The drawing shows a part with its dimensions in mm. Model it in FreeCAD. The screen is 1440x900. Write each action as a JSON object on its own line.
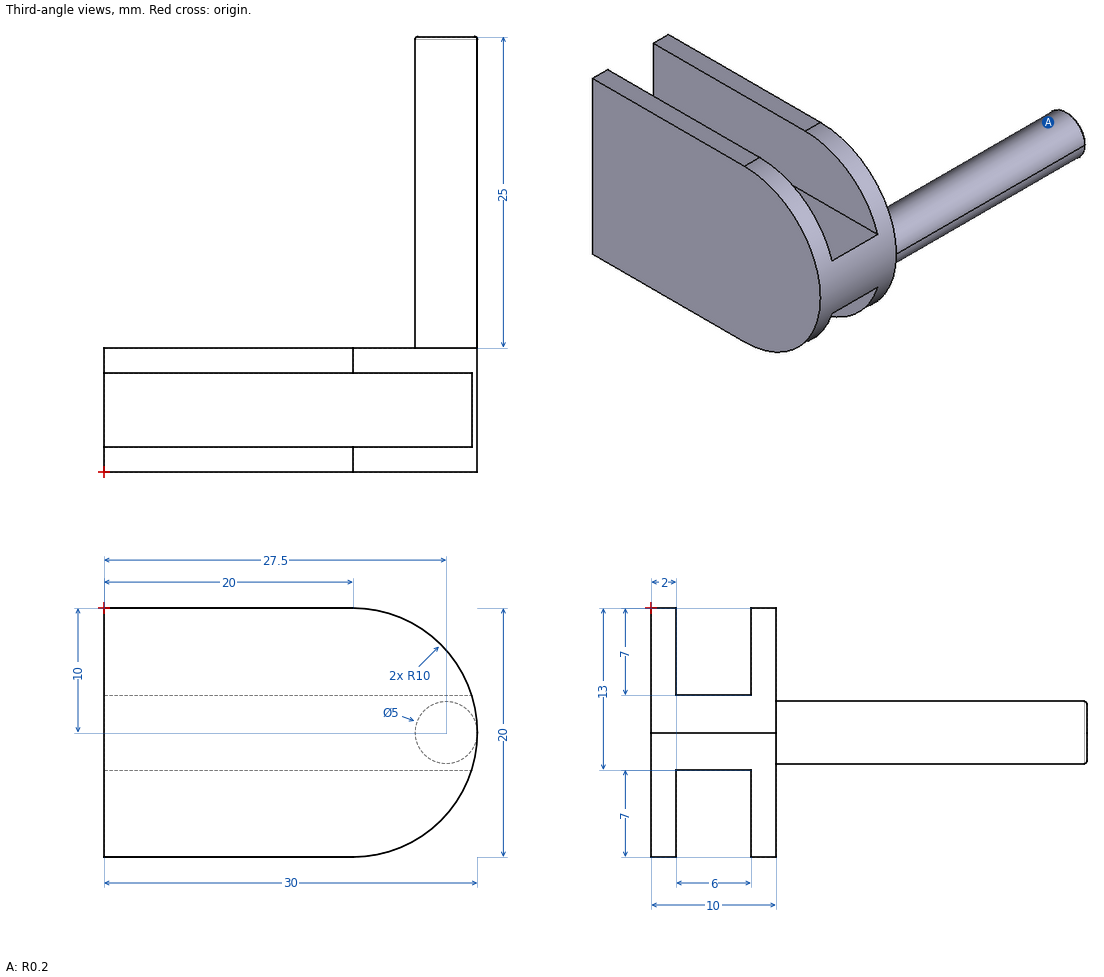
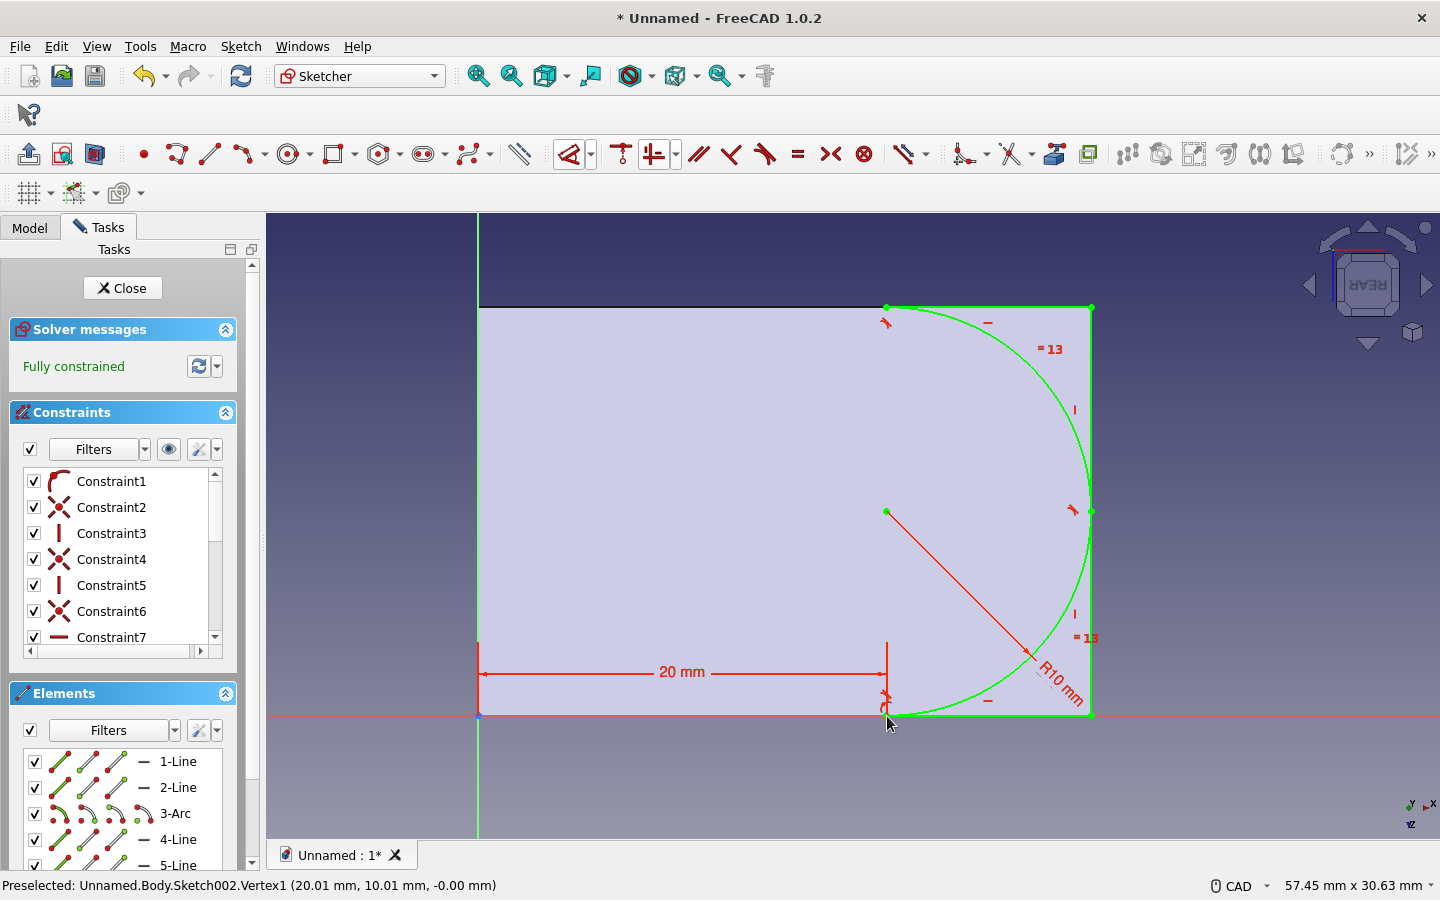
{"action": "left_click", "coordinate": [123, 288]}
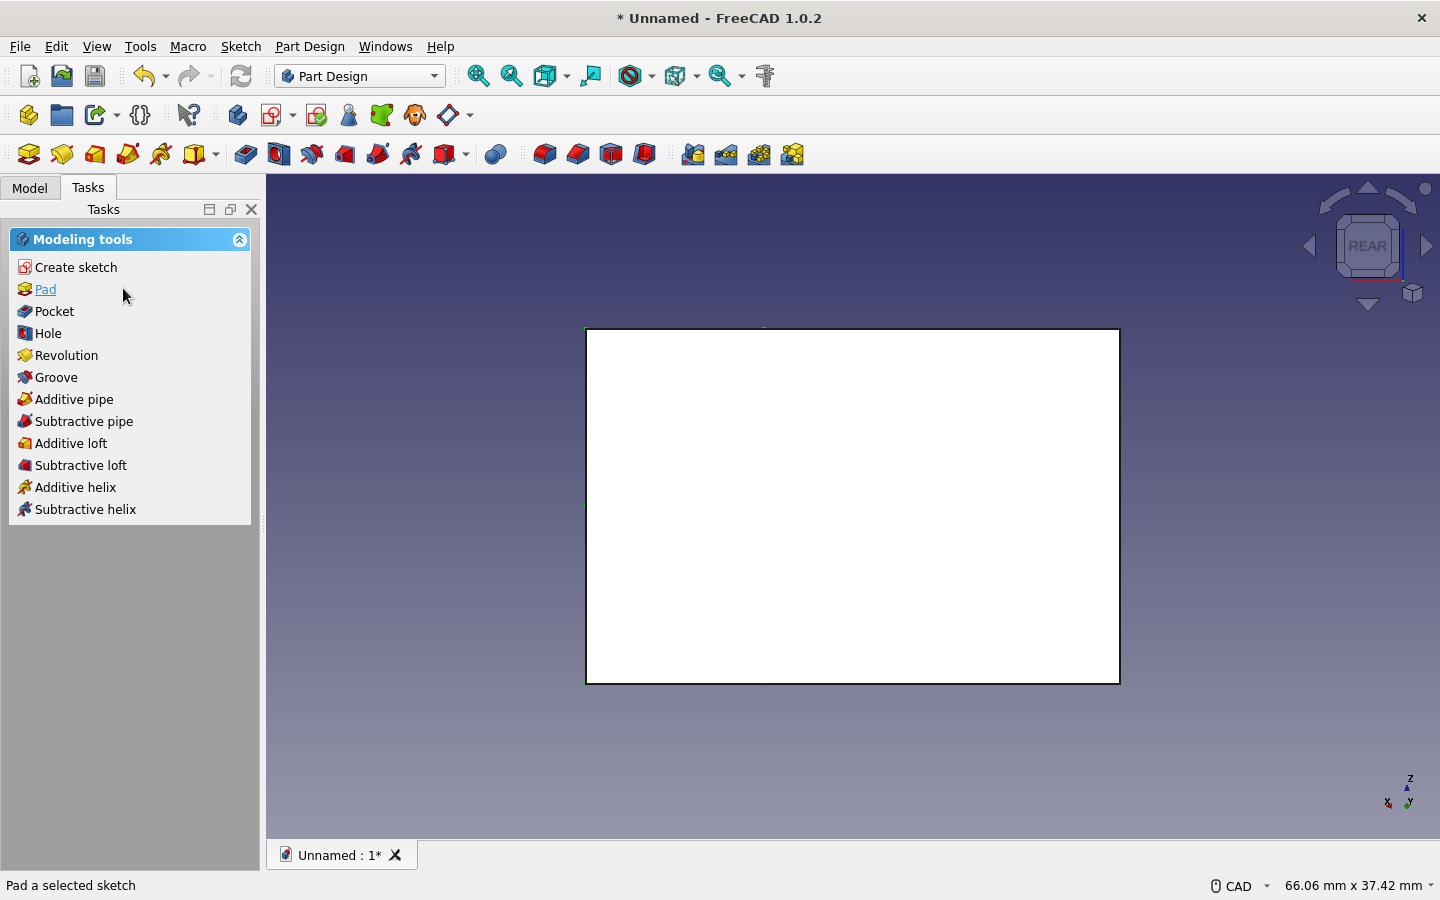
{"action": "left_click", "coordinate": [246, 154]}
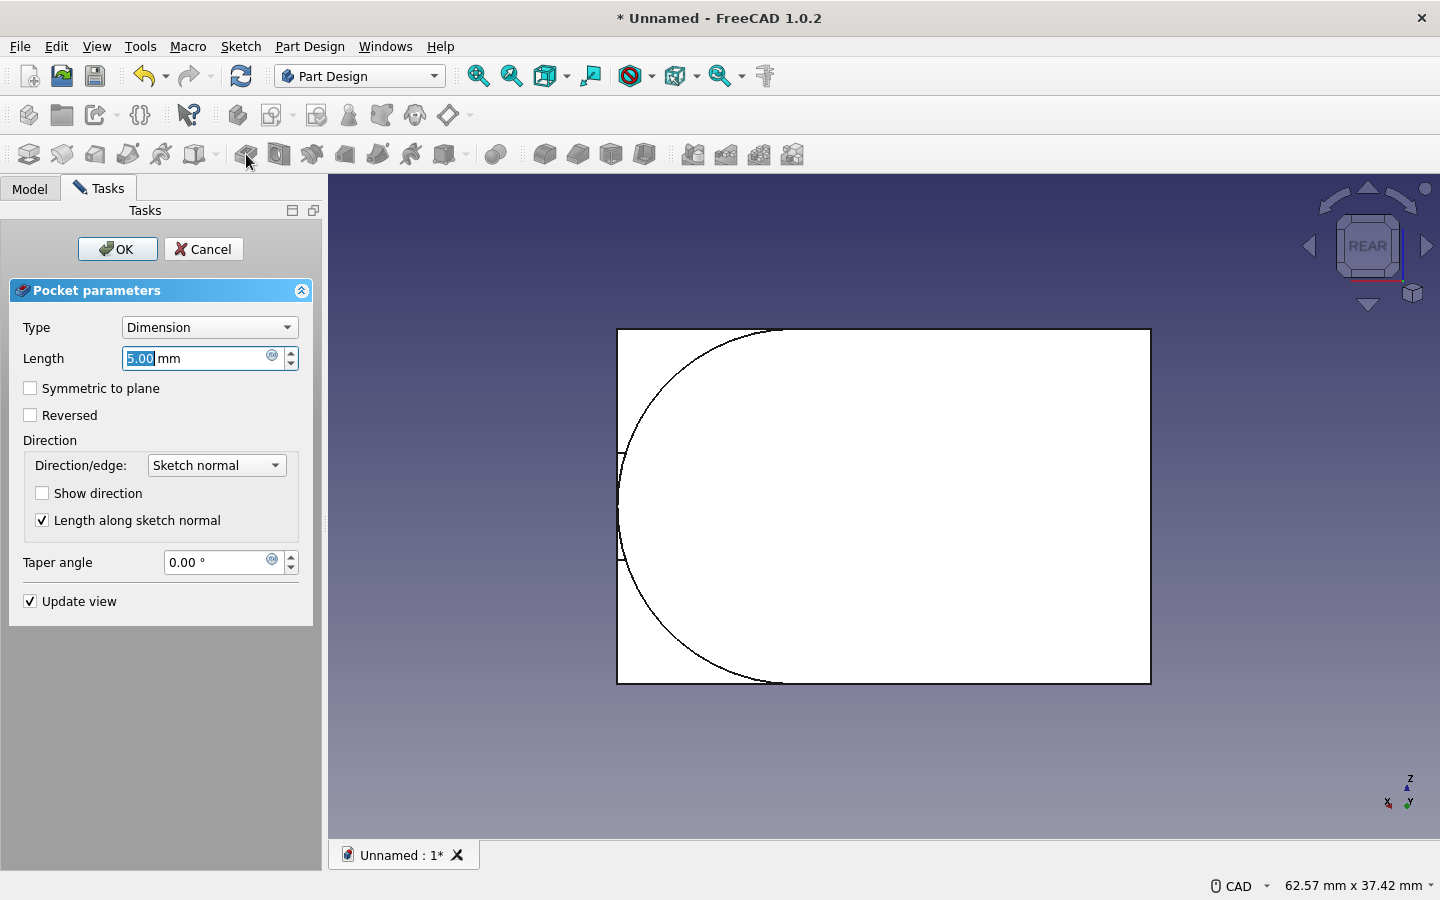
{"action": "left_click", "coordinate": [210, 328]}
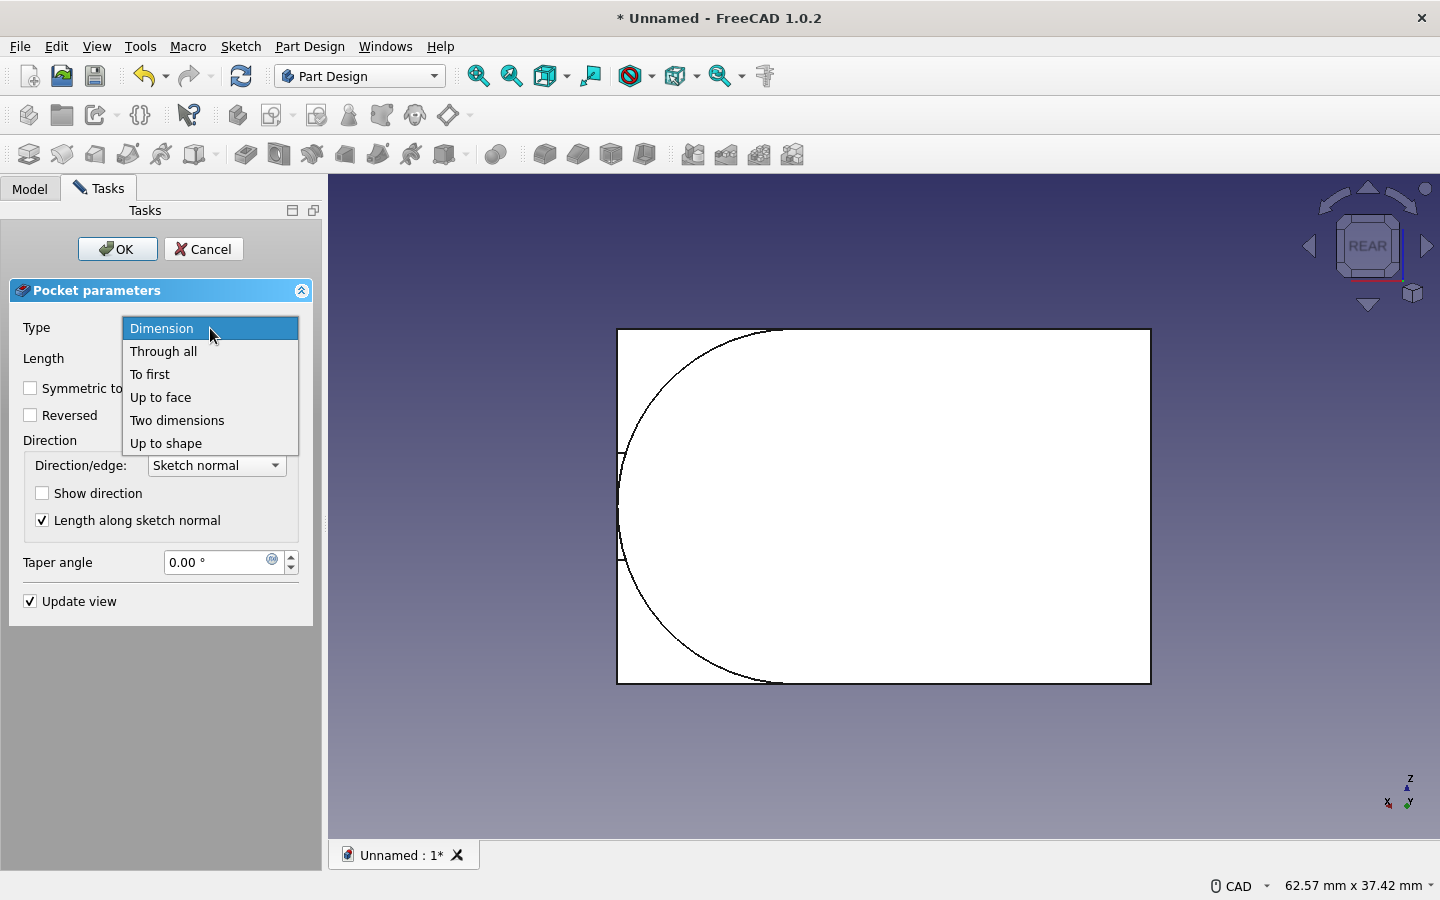
{"action": "left_click", "coordinate": [208, 352]}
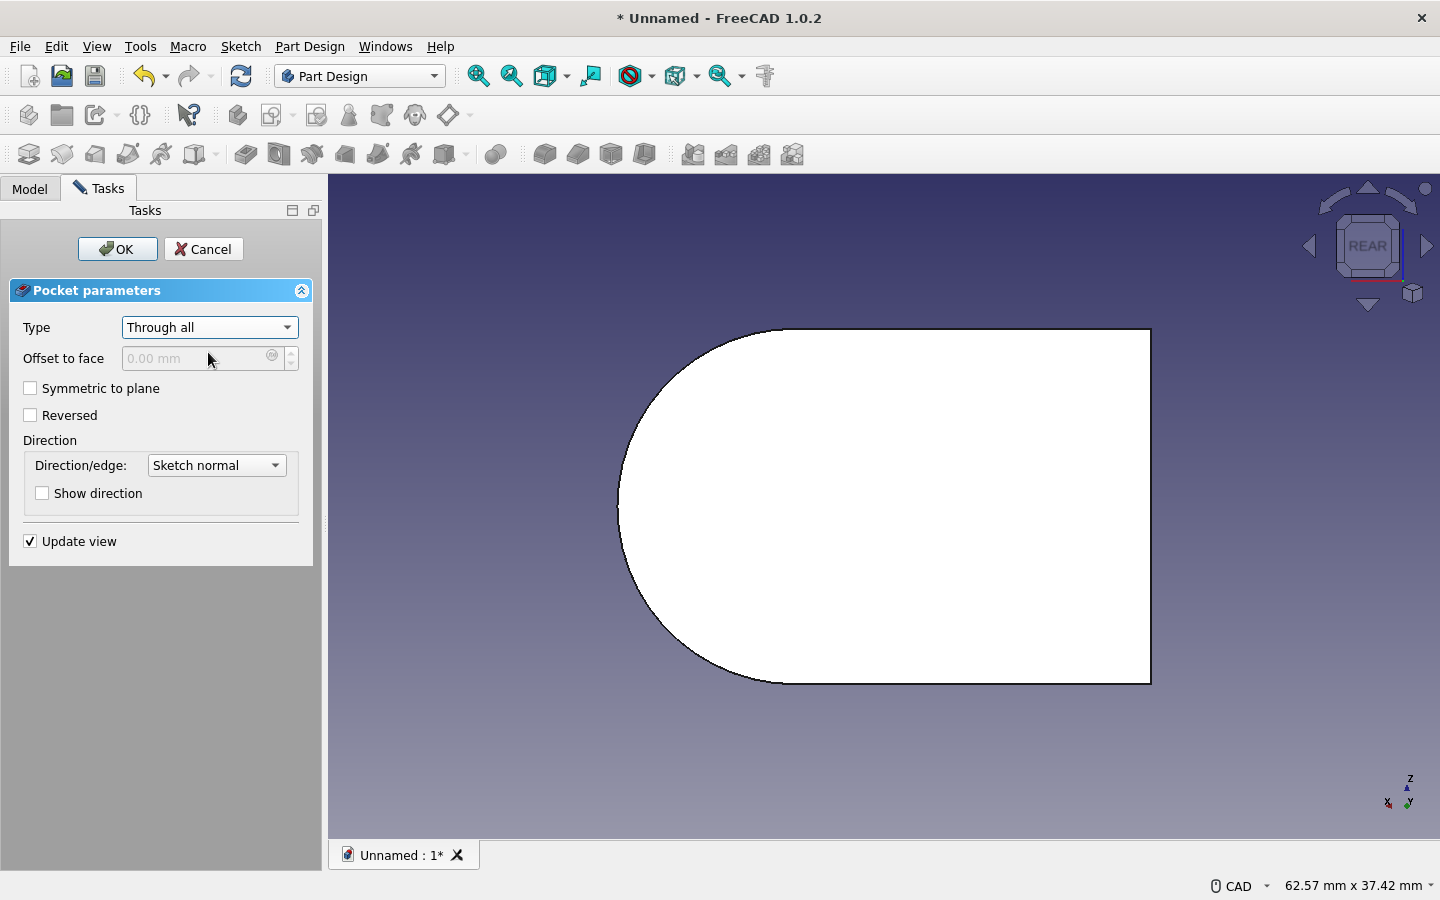
{"action": "left_click", "coordinate": [118, 249]}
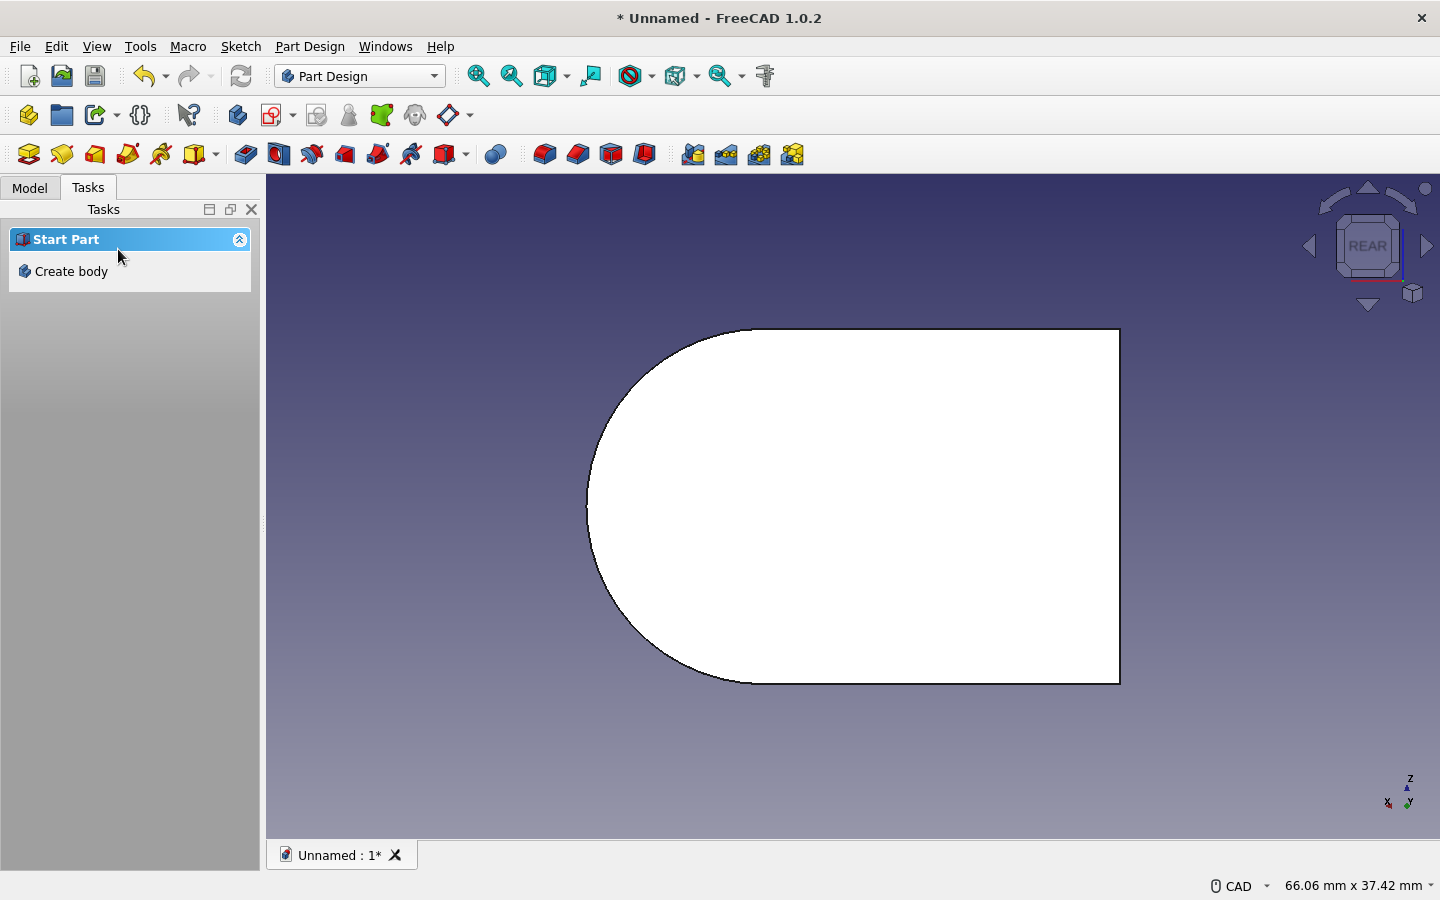
{"action": "left_click", "coordinate": [777, 506]}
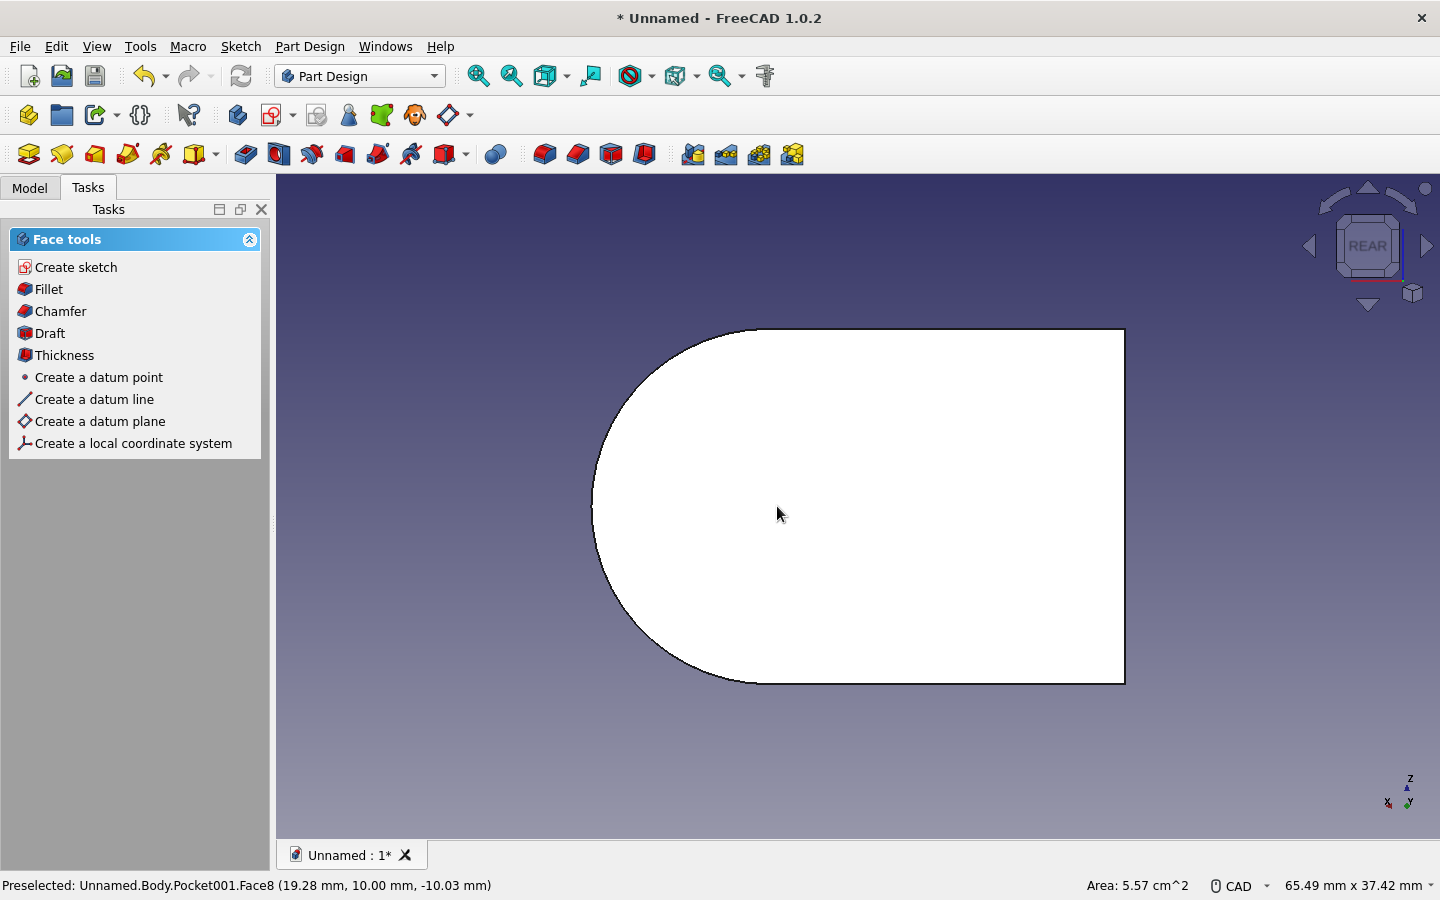
{"action": "left_click", "coordinate": [270, 116]}